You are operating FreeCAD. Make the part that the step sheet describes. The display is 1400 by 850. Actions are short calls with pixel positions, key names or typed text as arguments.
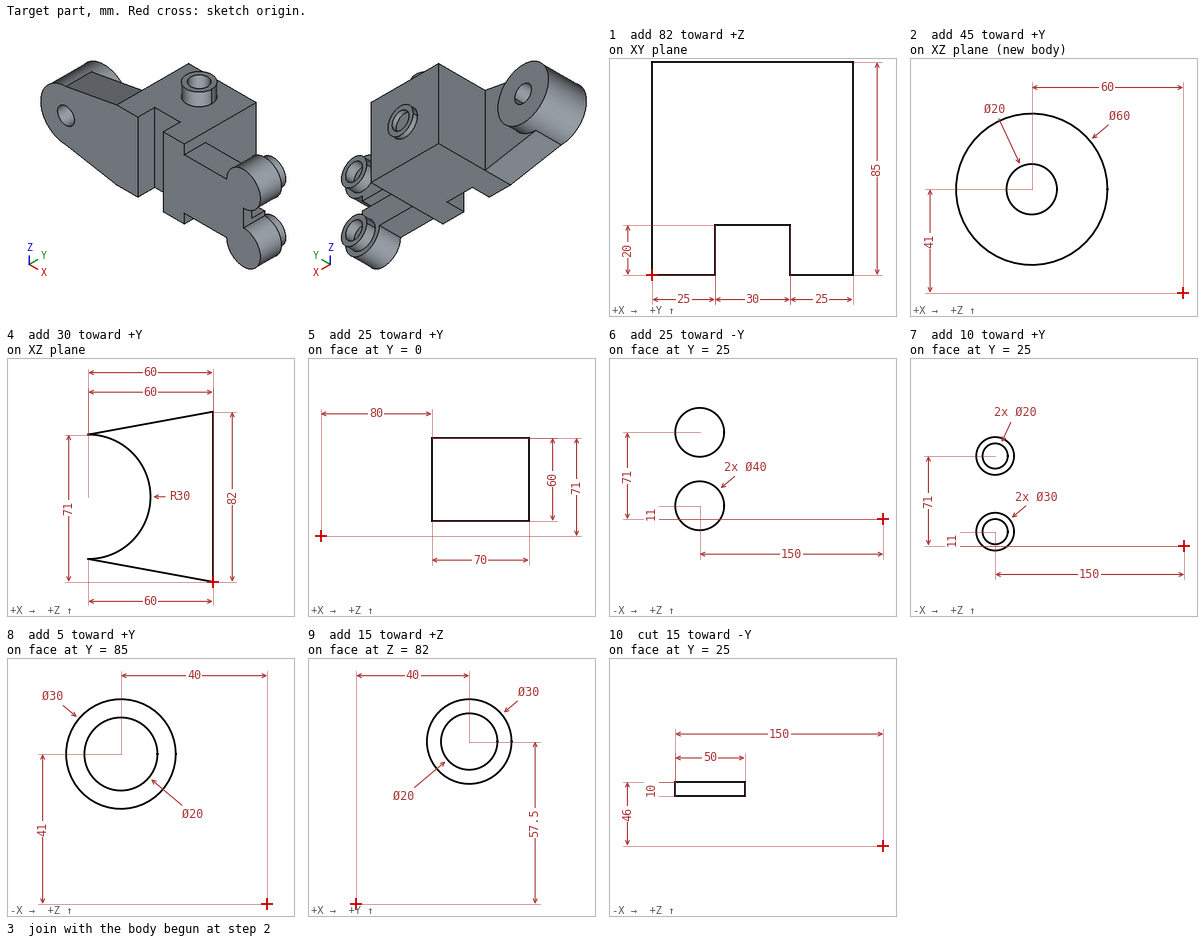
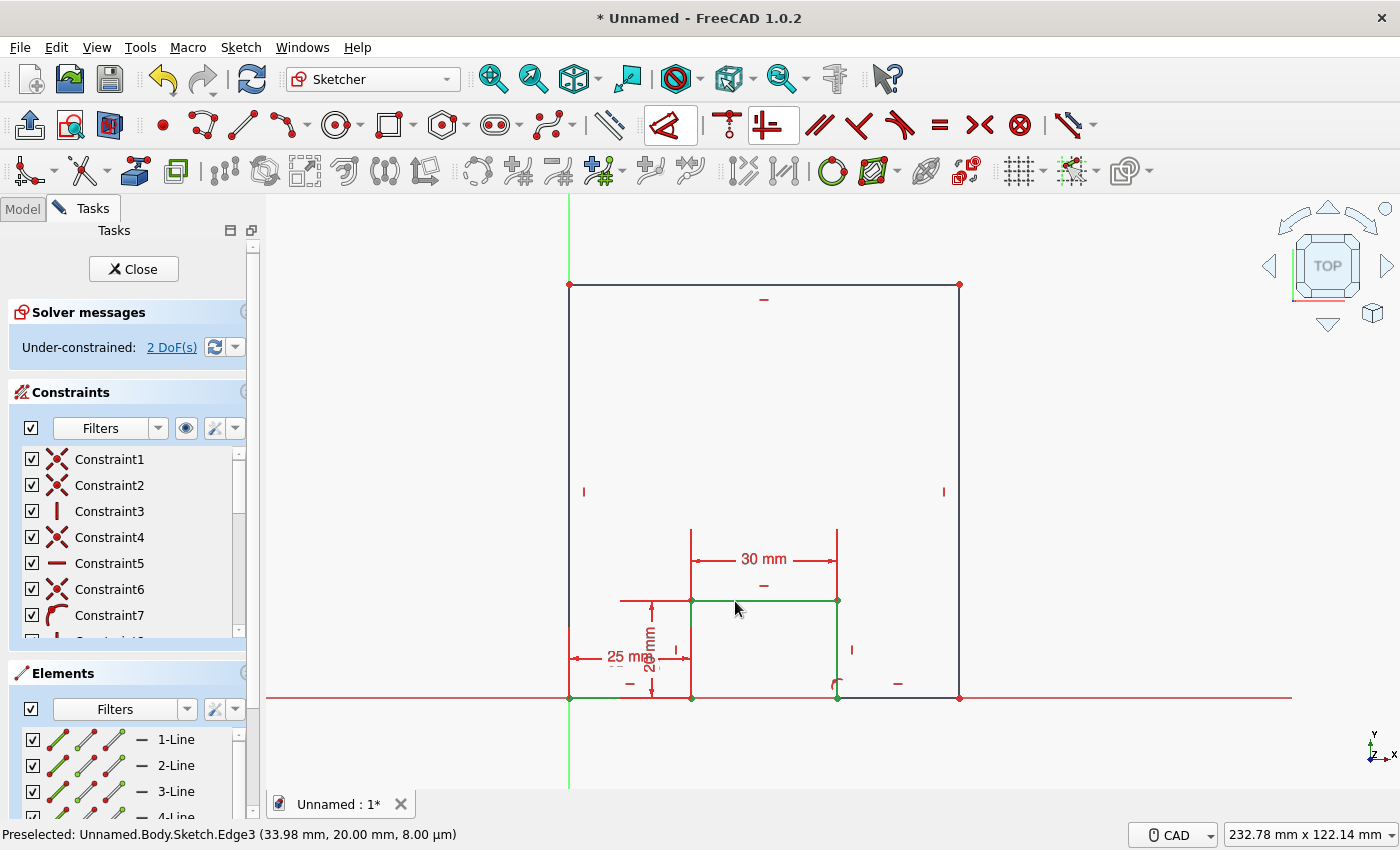
click(874, 698)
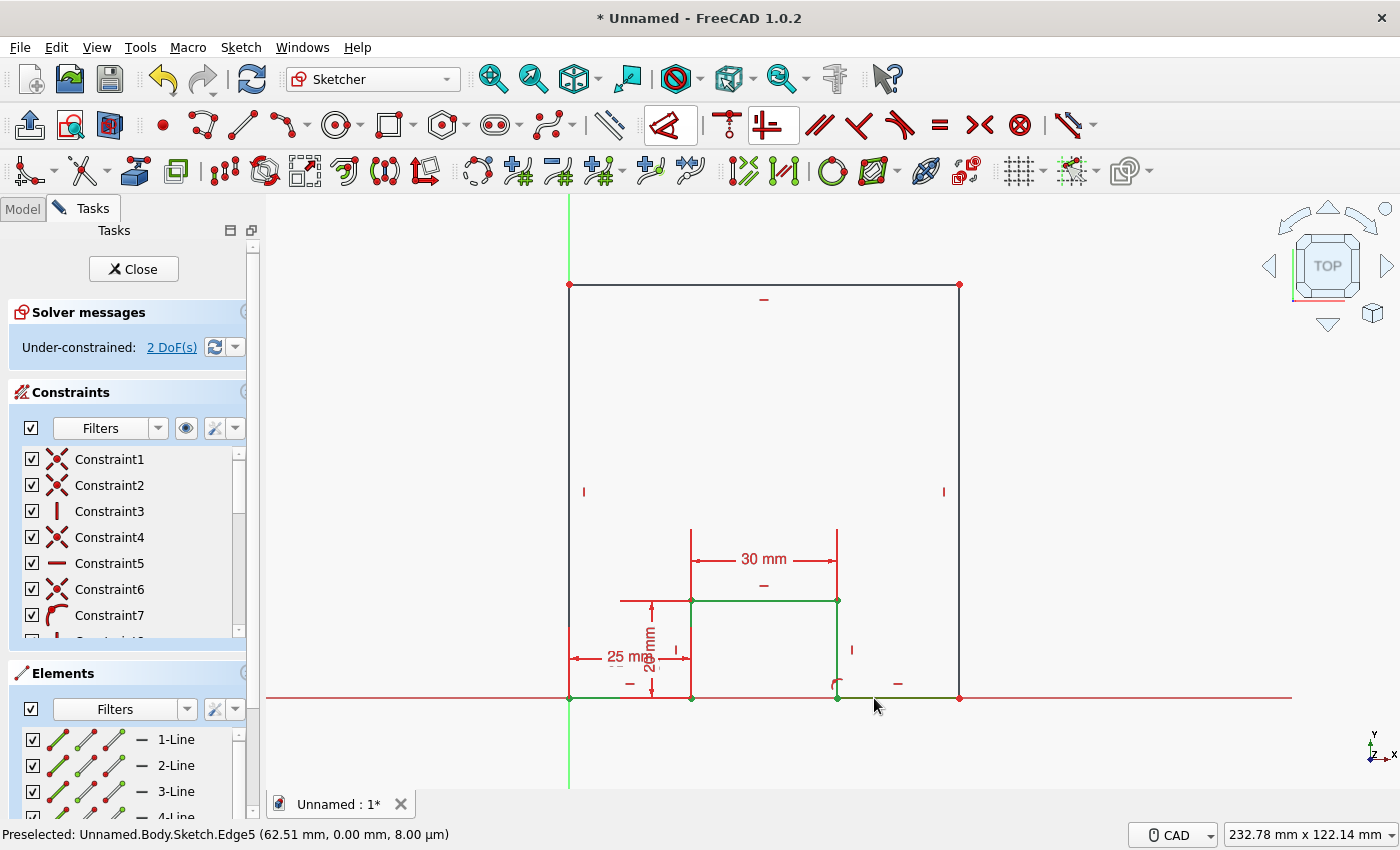
click(692, 126)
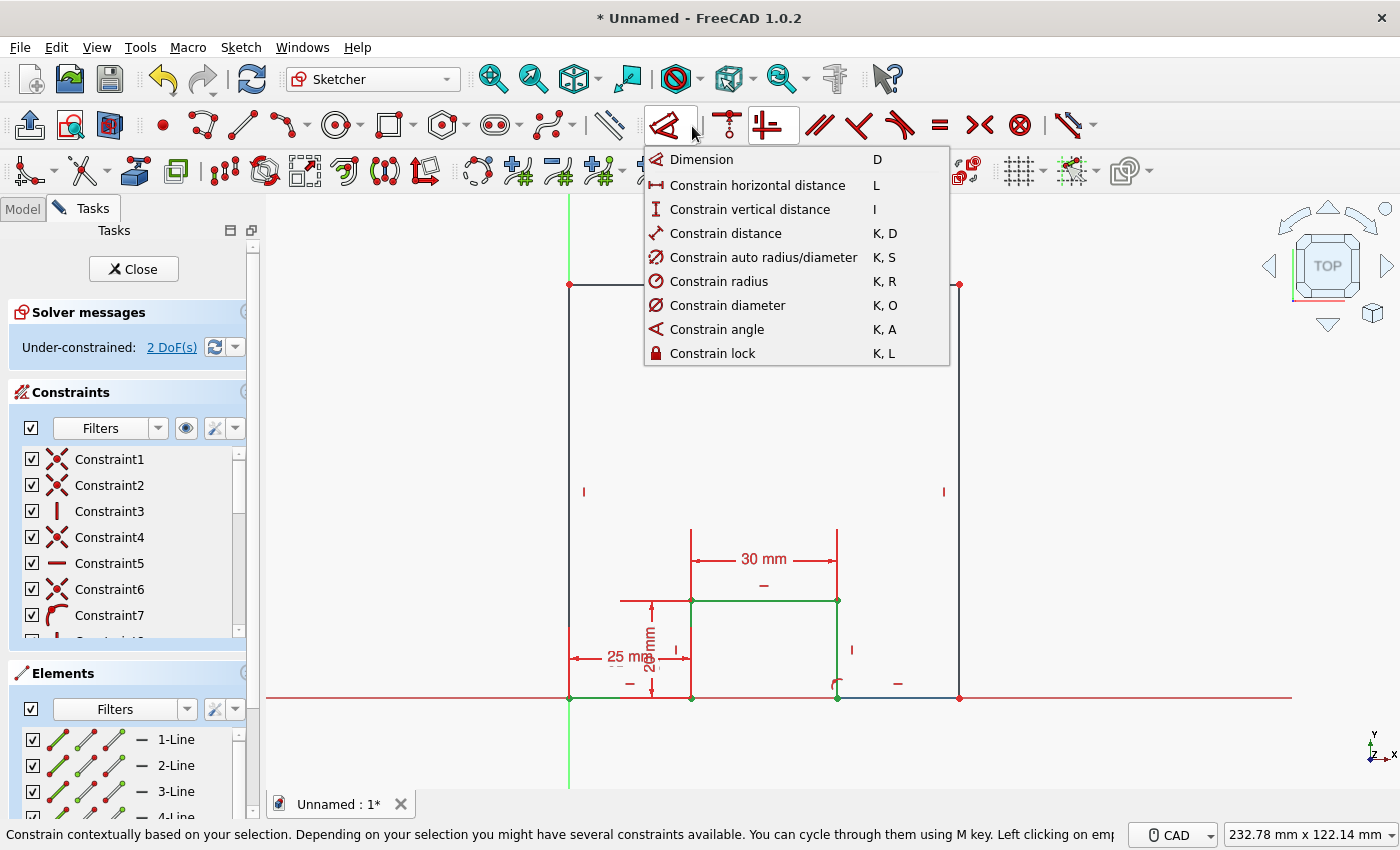
click(797, 185)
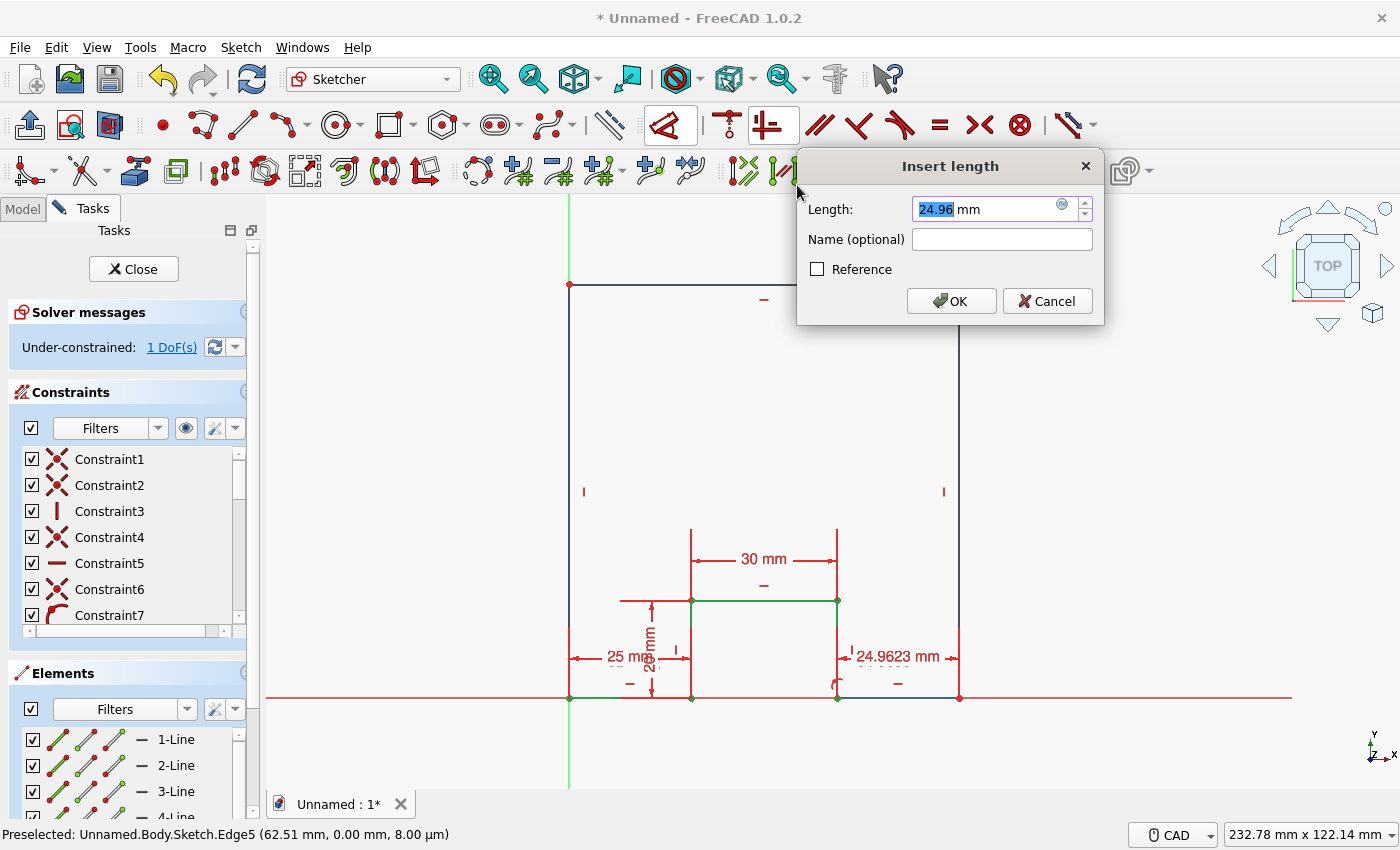
text(25)
key(Return)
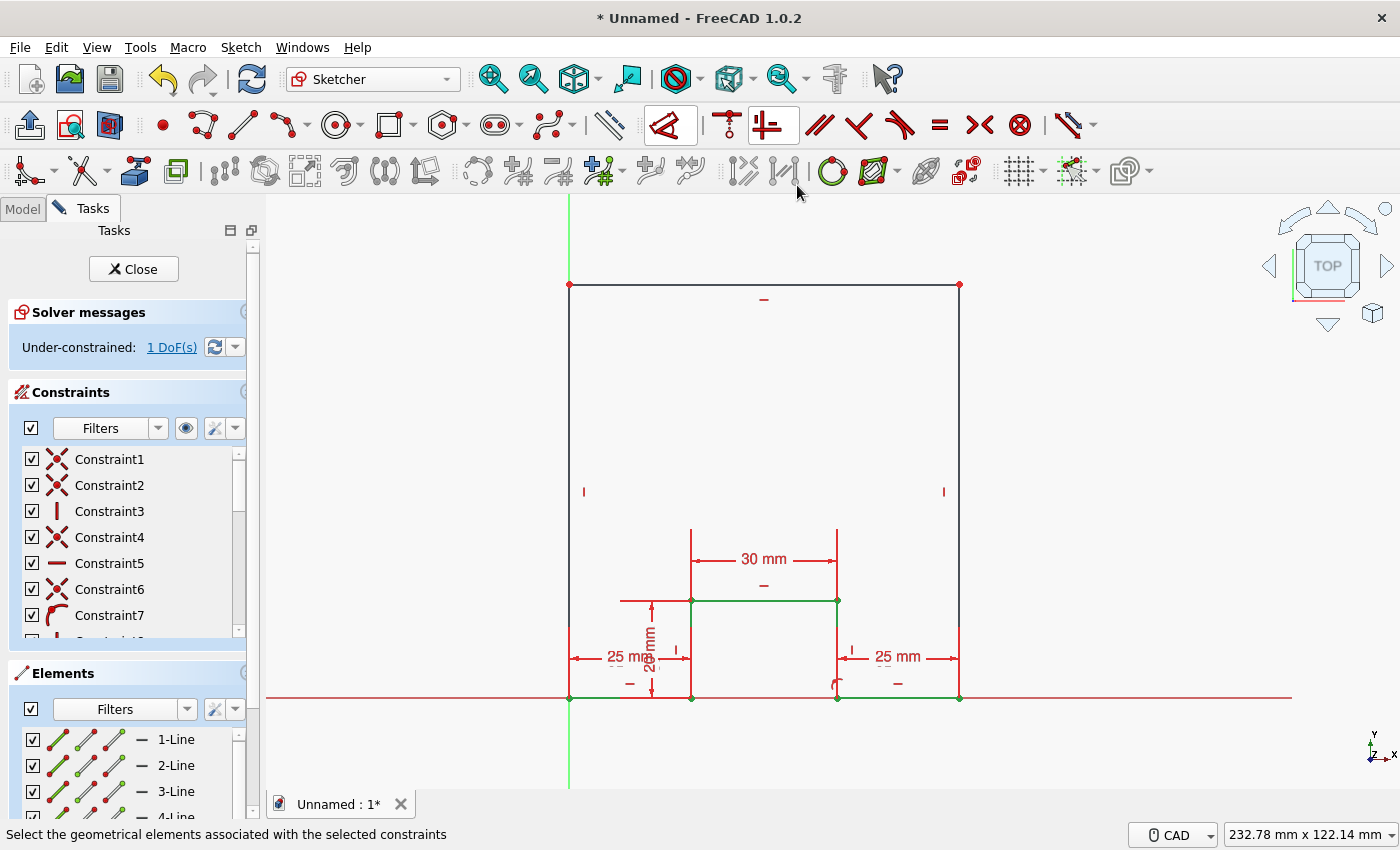
click(959, 574)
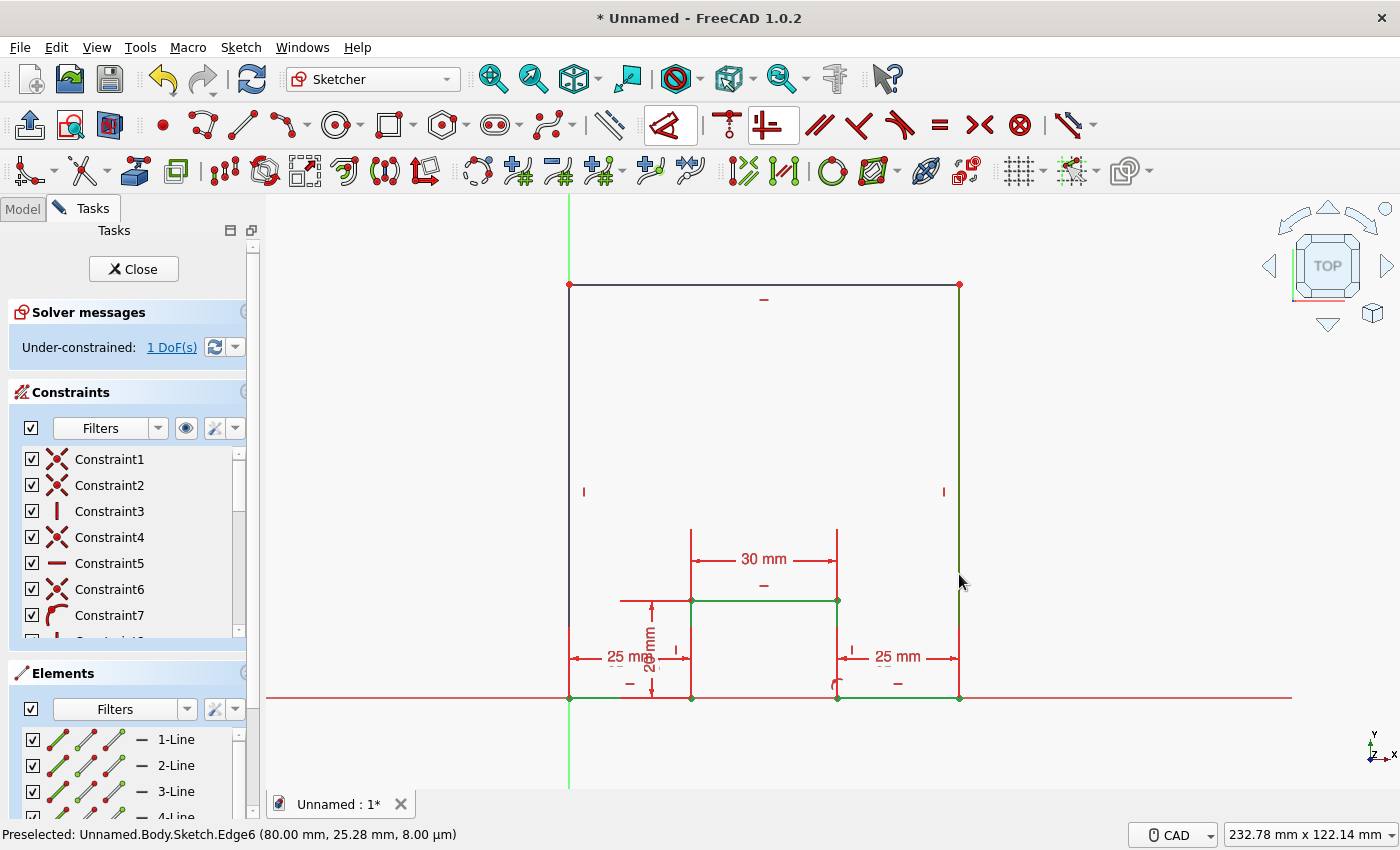
key(i)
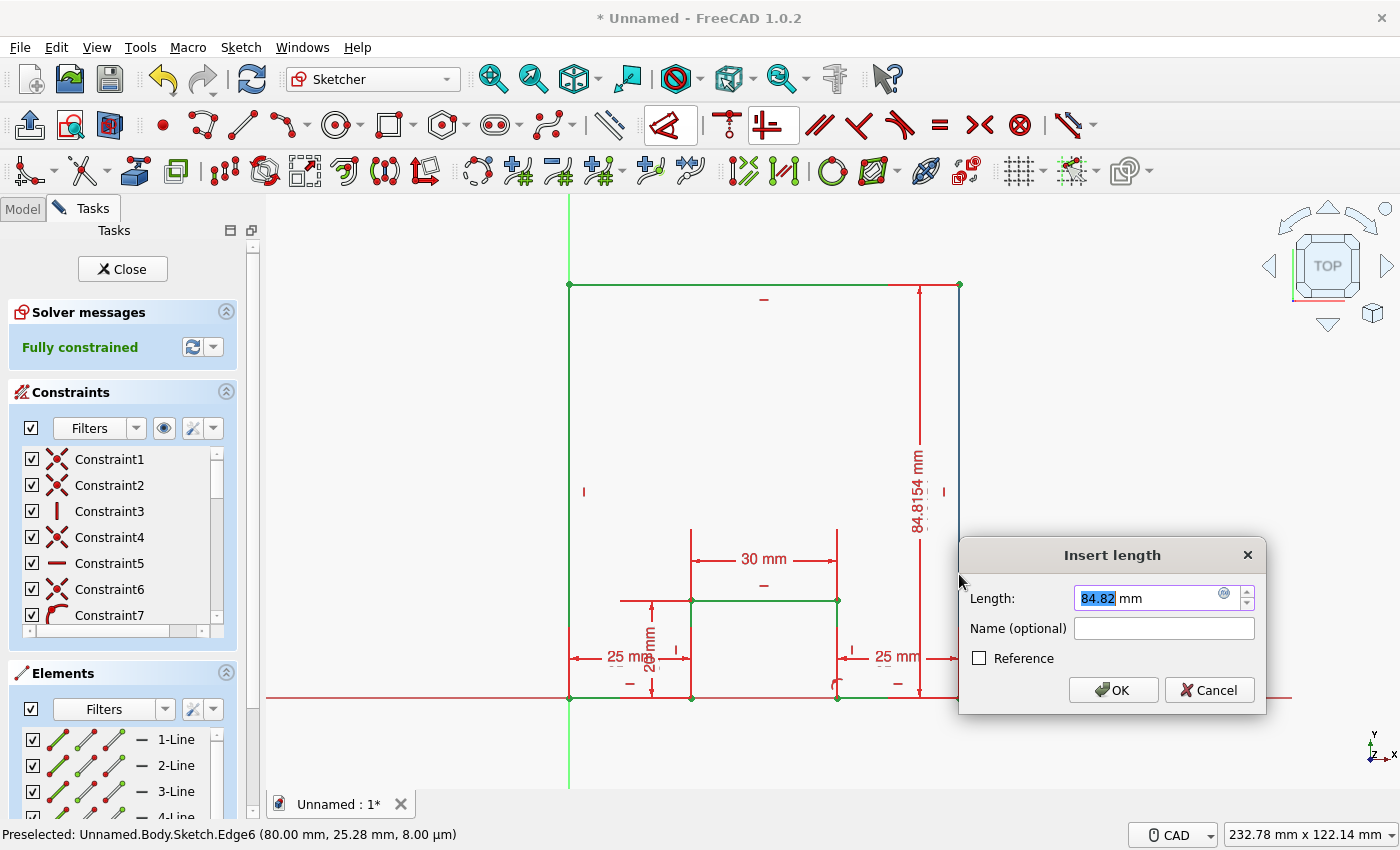
text(85)
key(Return)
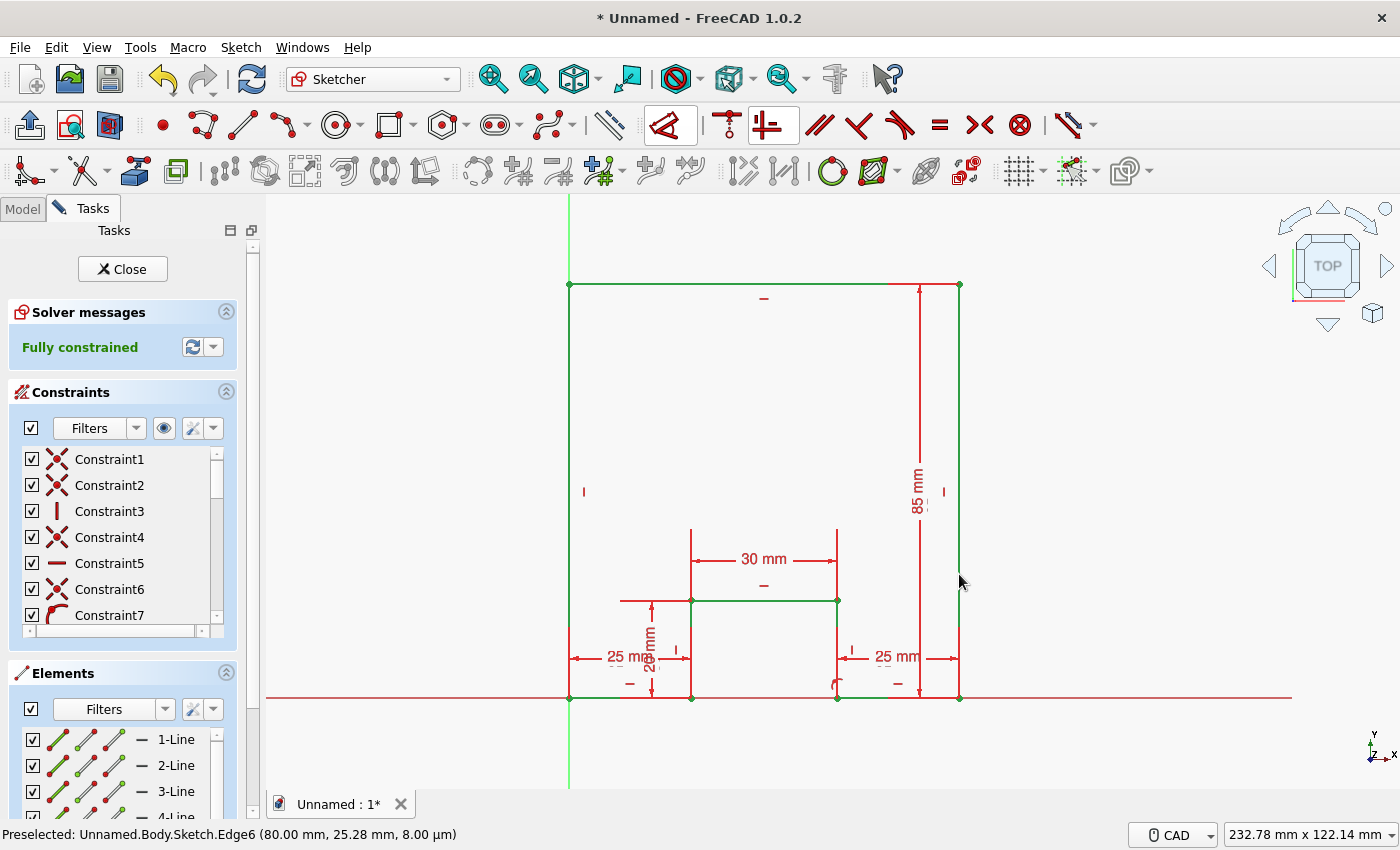
click(123, 269)